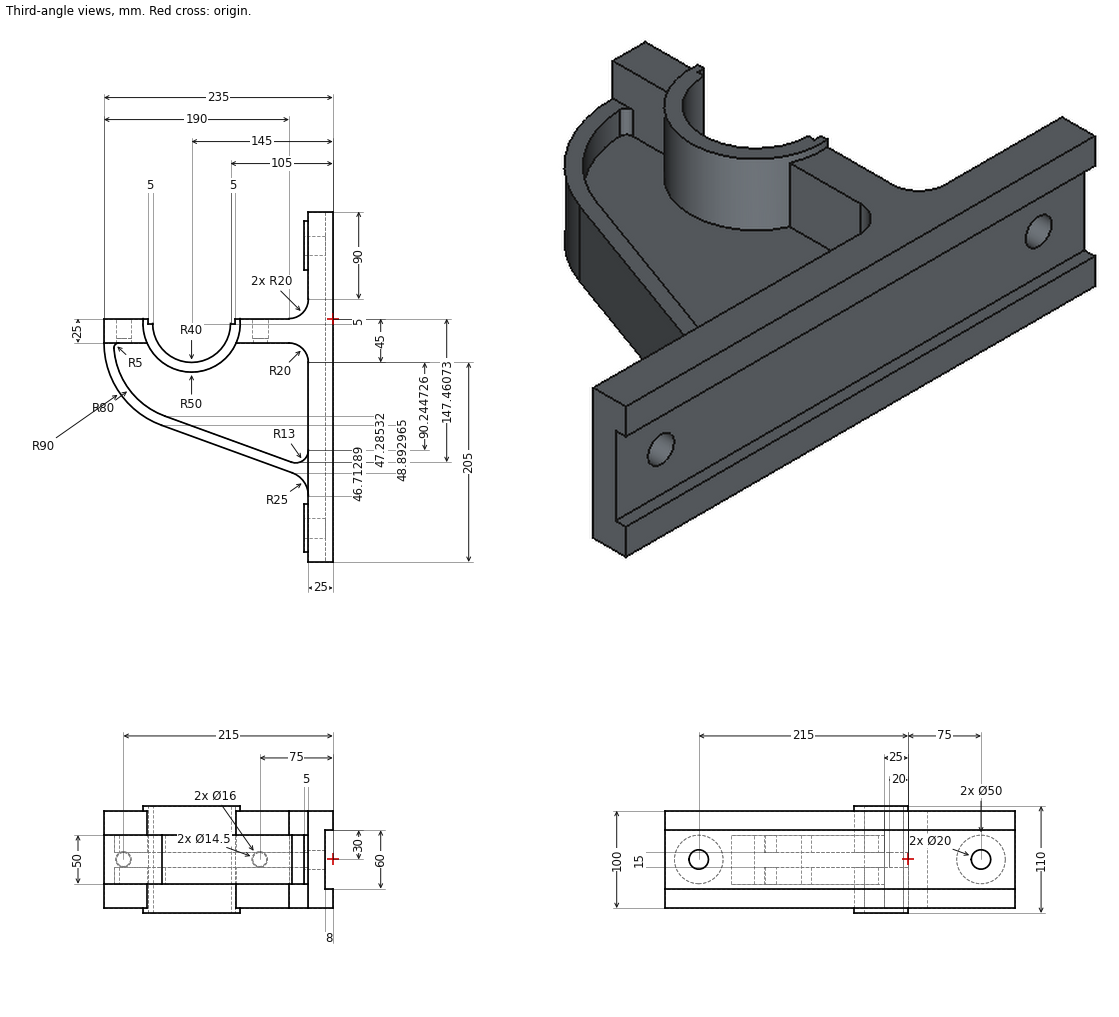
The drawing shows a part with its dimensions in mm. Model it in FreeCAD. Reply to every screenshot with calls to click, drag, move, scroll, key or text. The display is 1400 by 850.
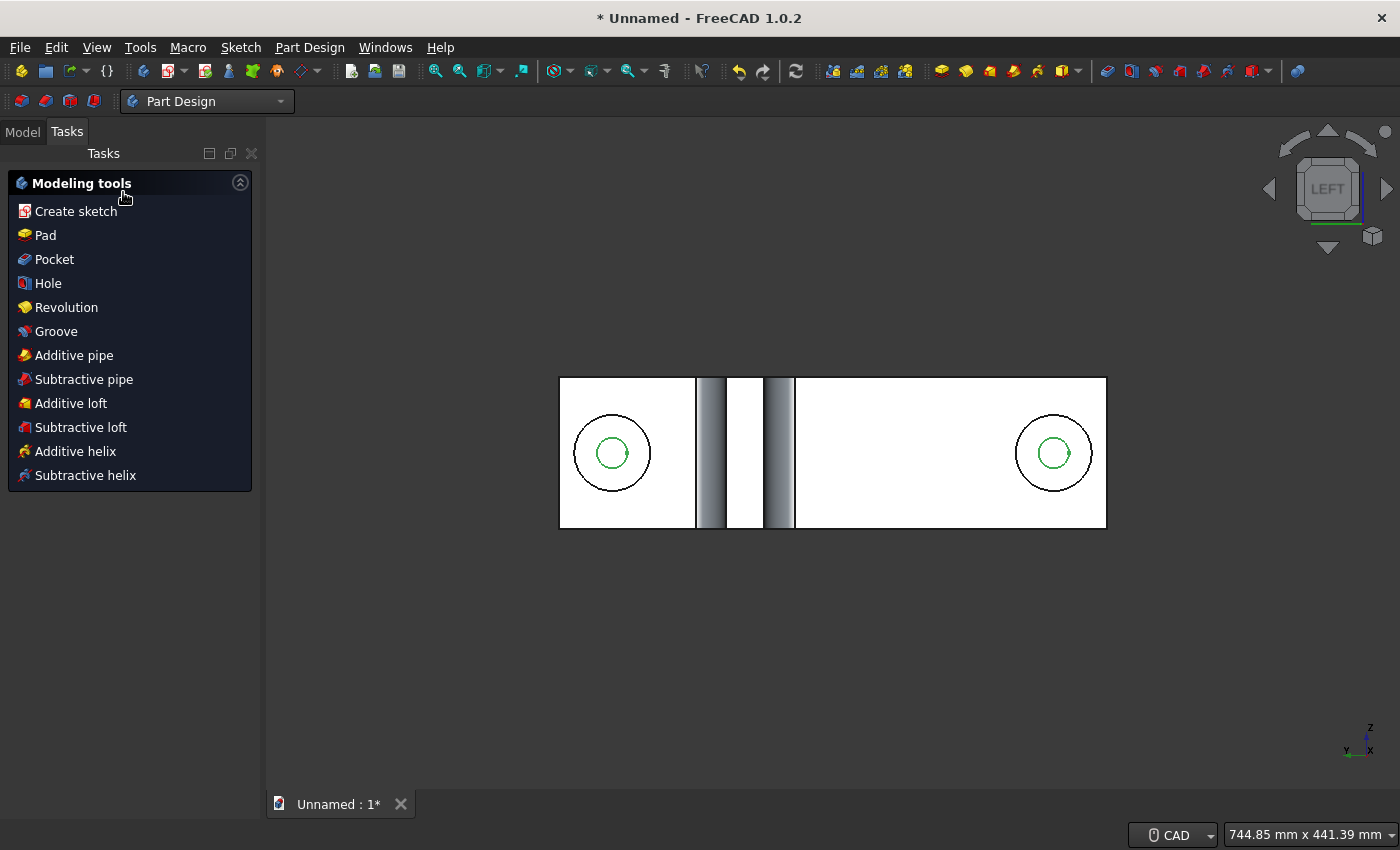
click(1108, 72)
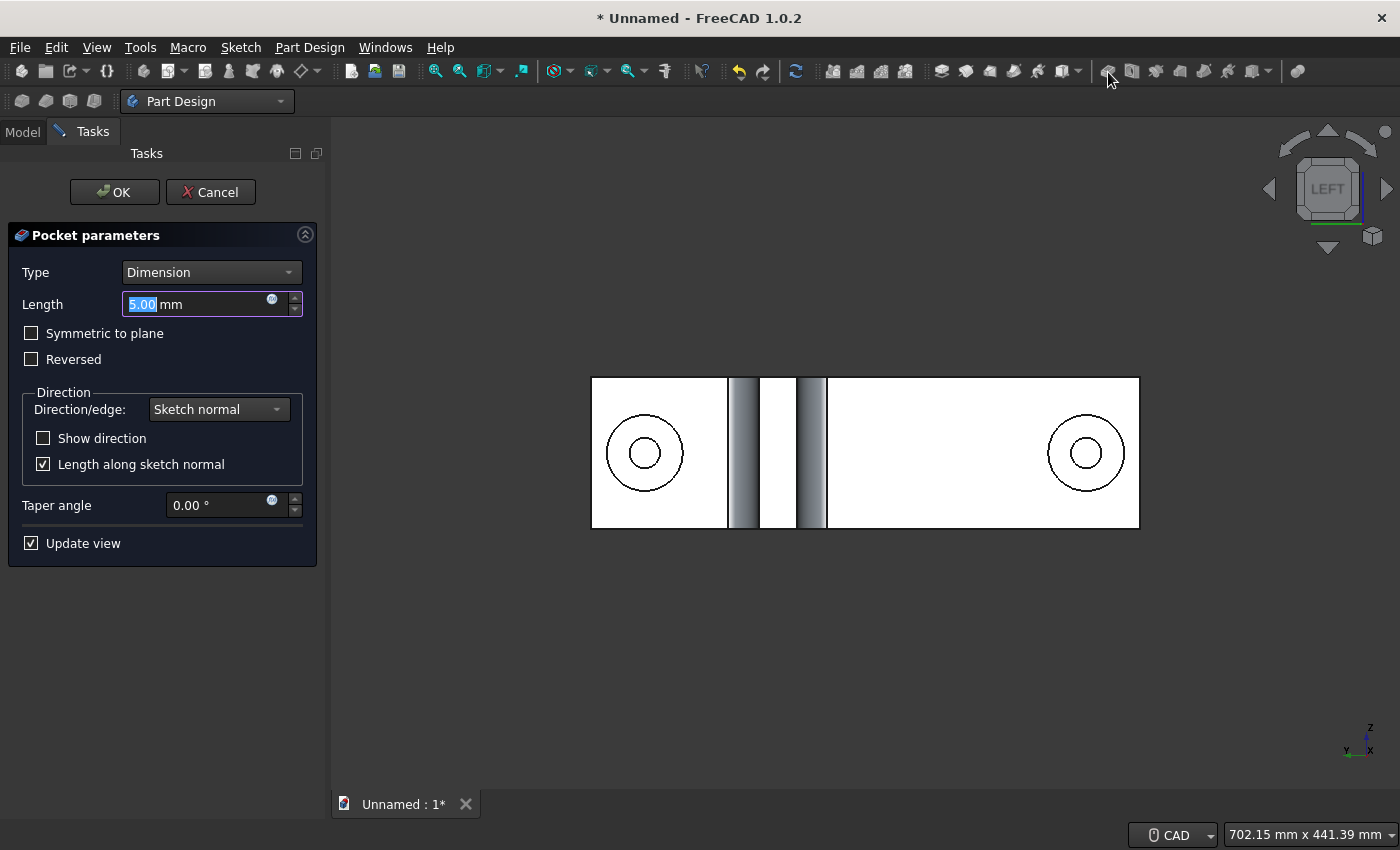
click(212, 272)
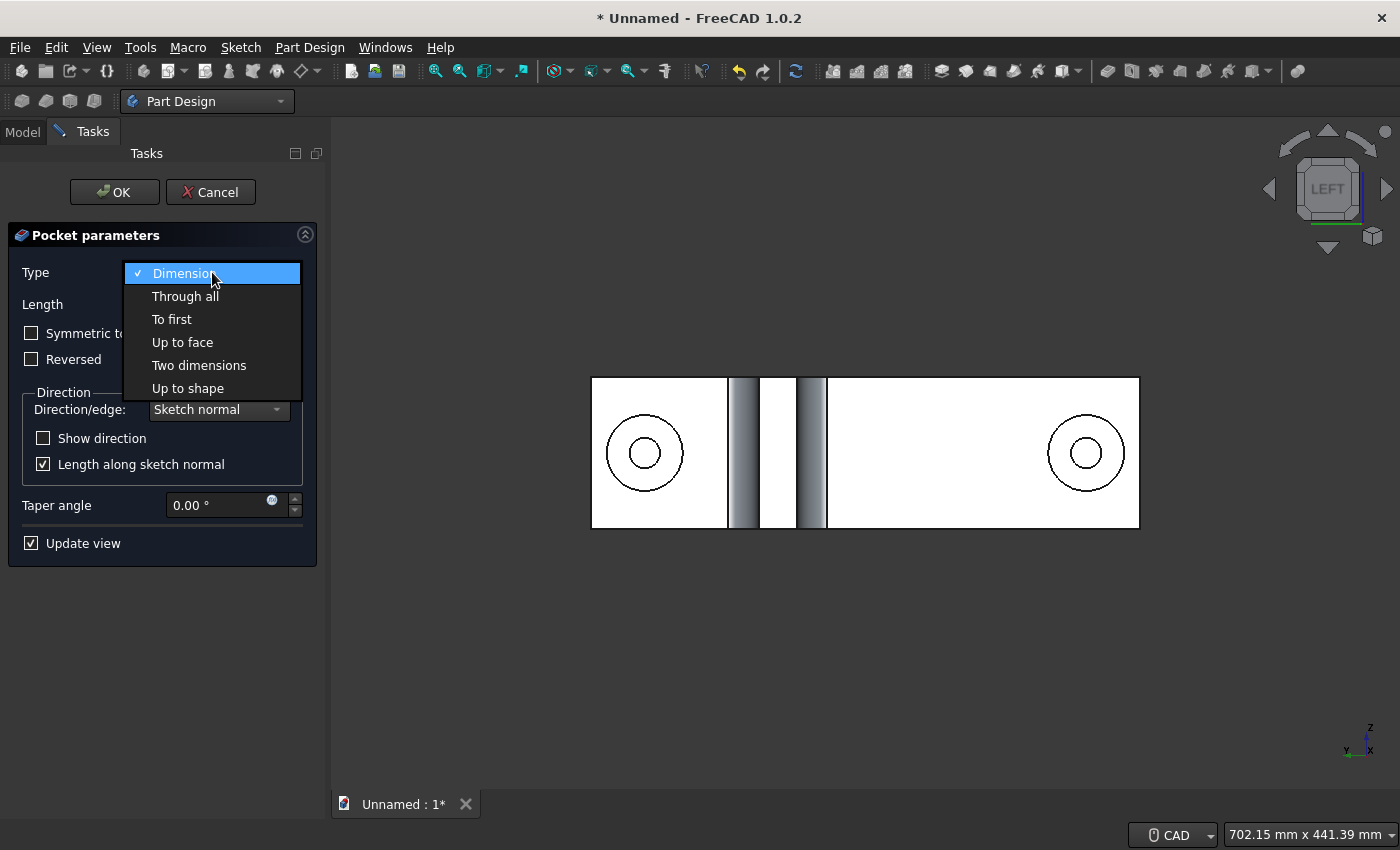
click(212, 296)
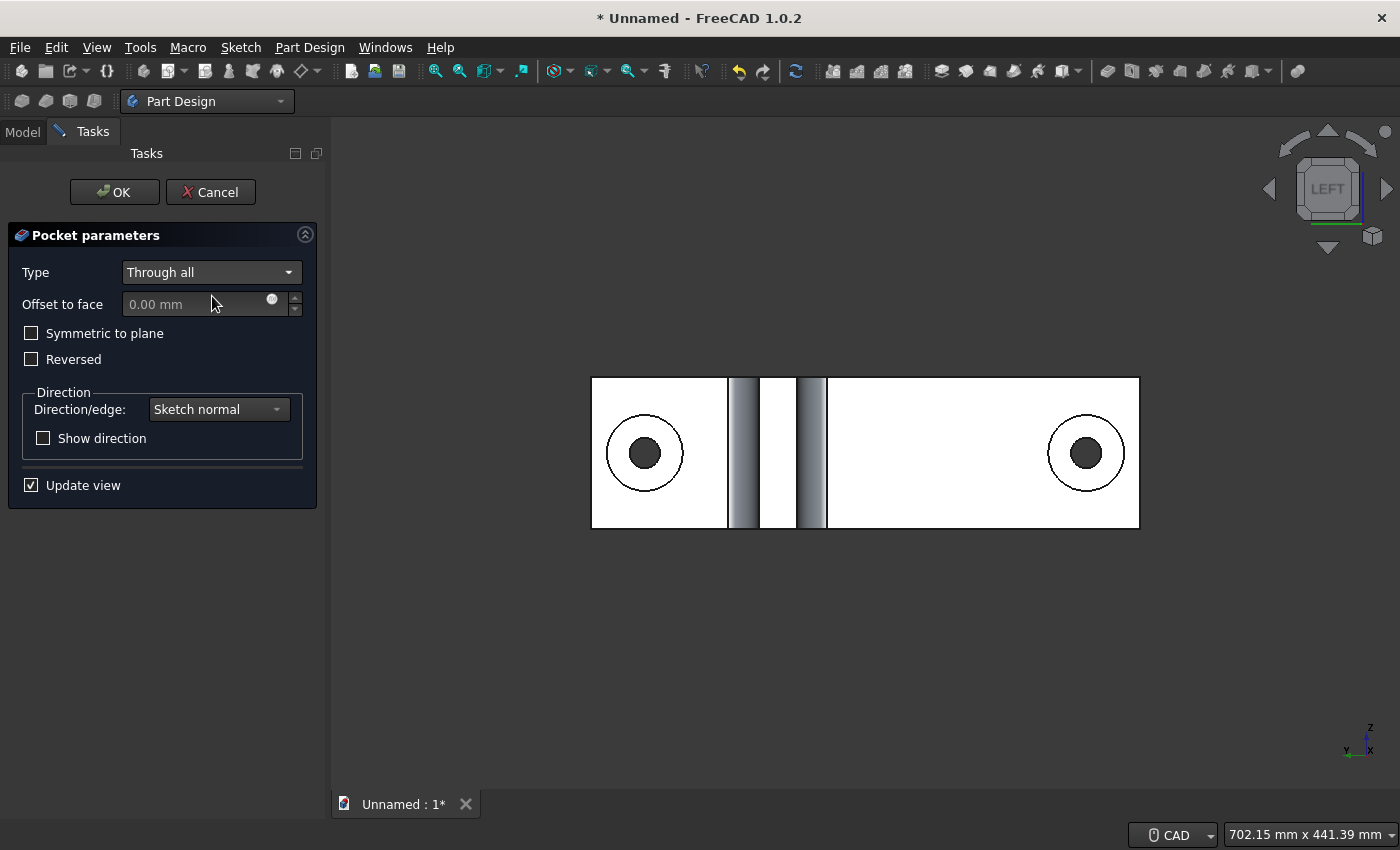
click(115, 192)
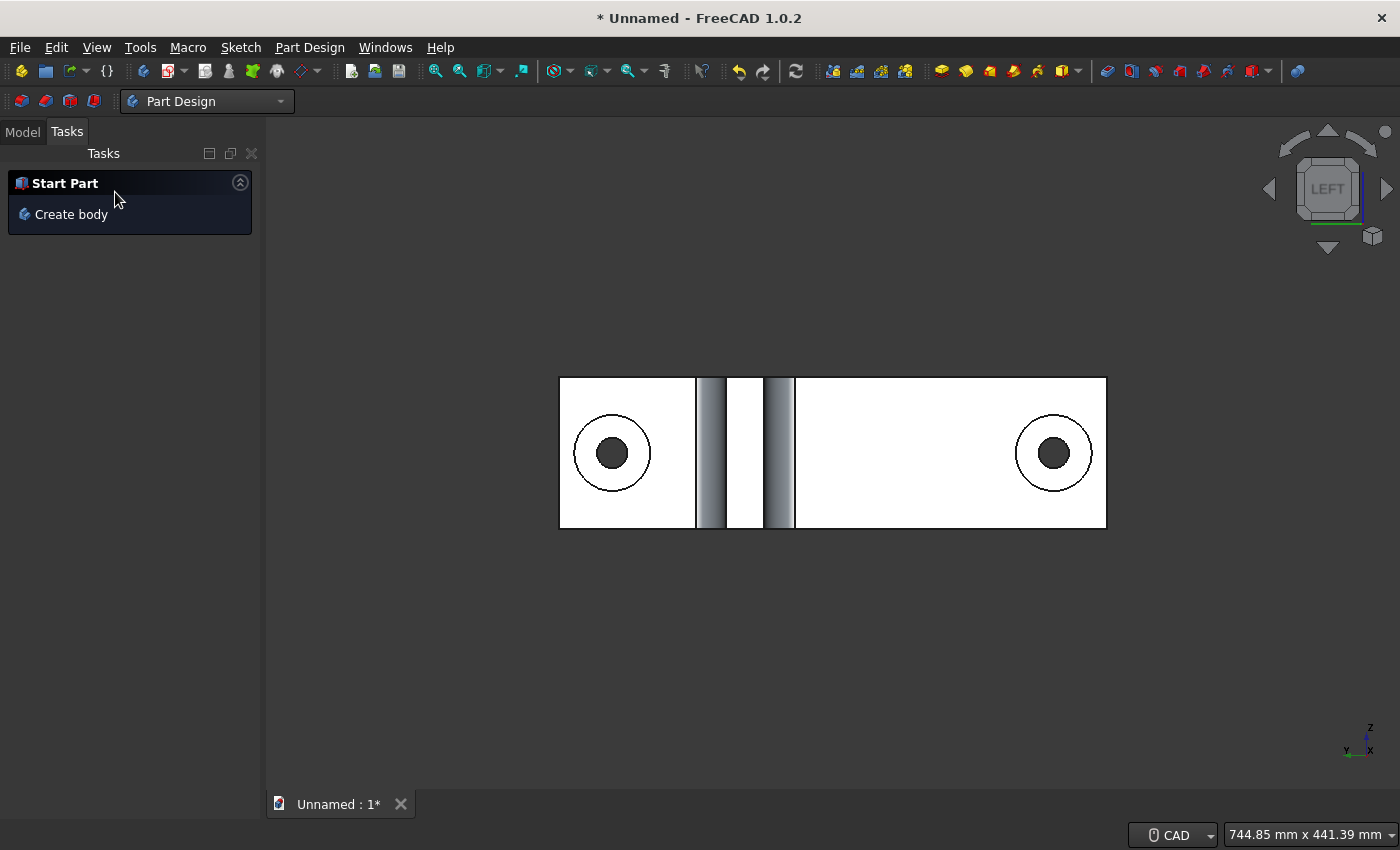
click(168, 72)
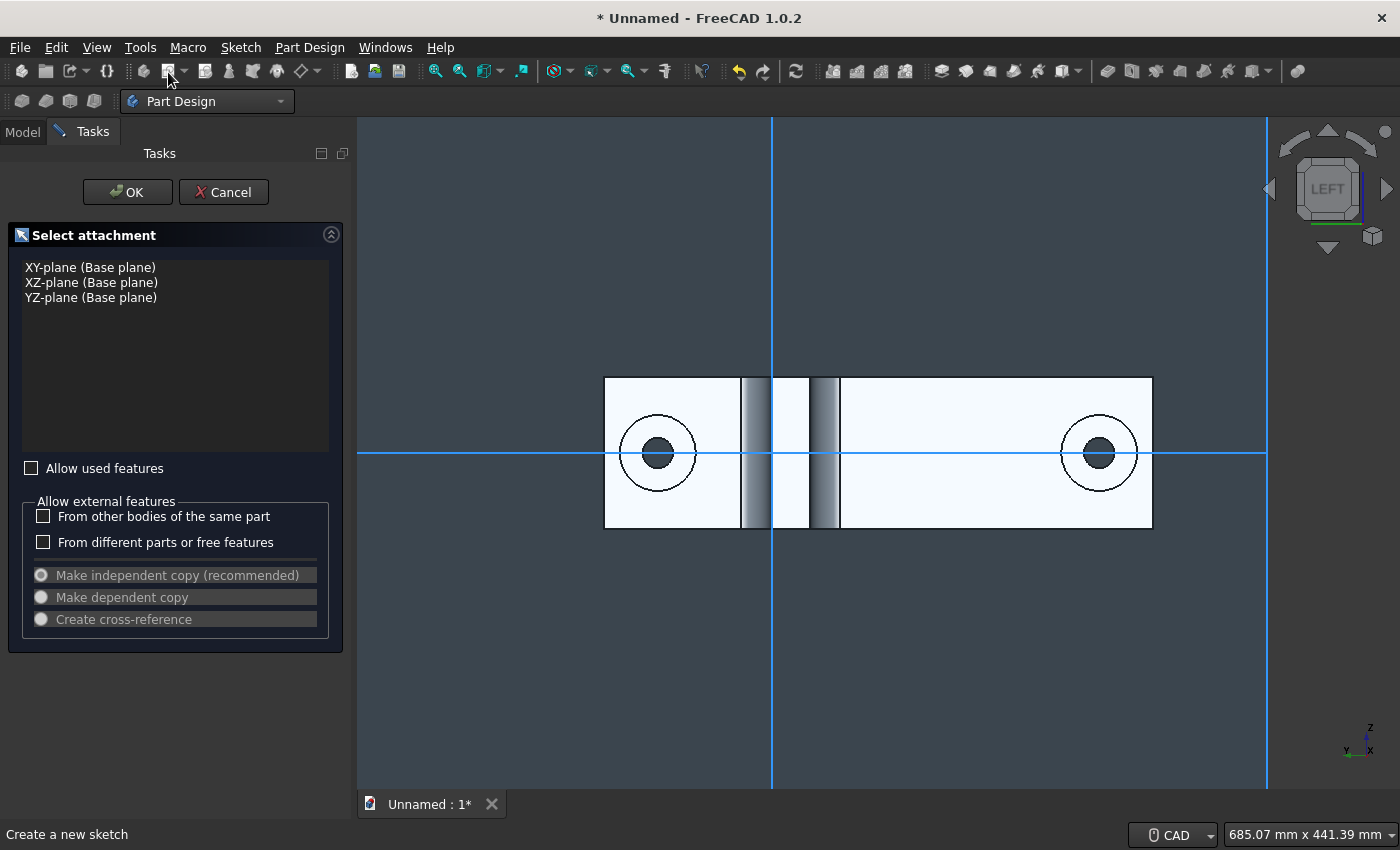
click(82, 282)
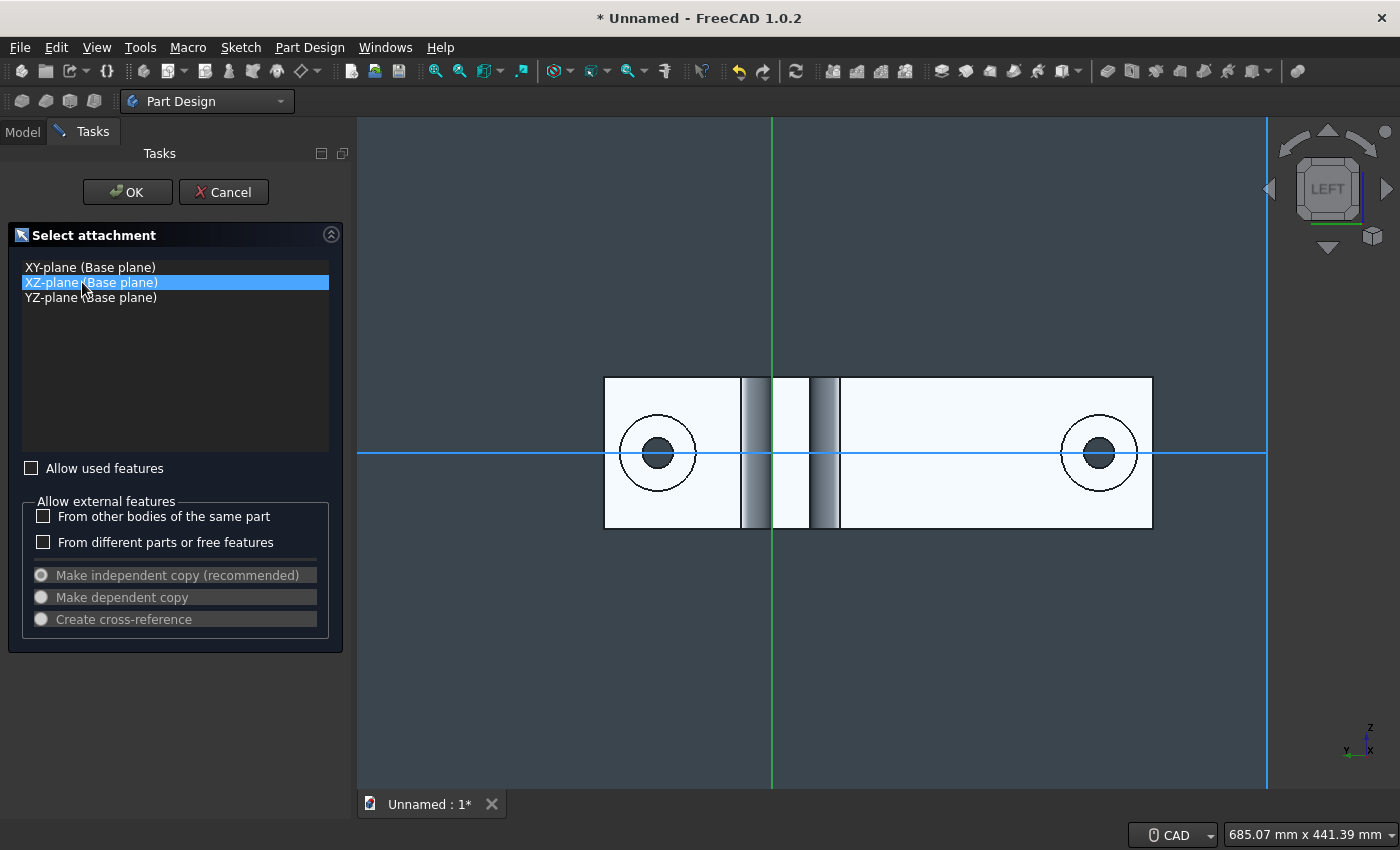
click(128, 192)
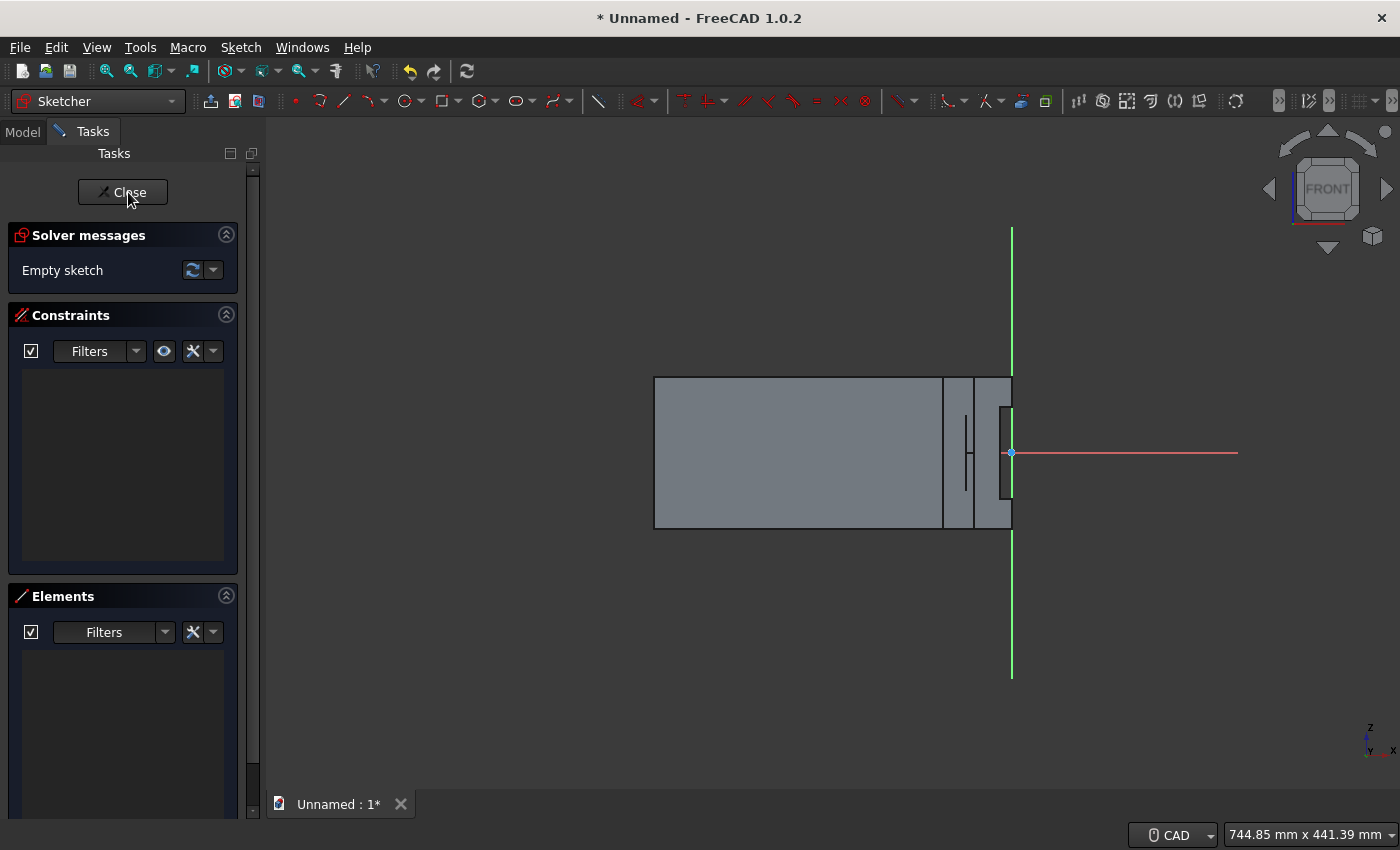
click(260, 102)